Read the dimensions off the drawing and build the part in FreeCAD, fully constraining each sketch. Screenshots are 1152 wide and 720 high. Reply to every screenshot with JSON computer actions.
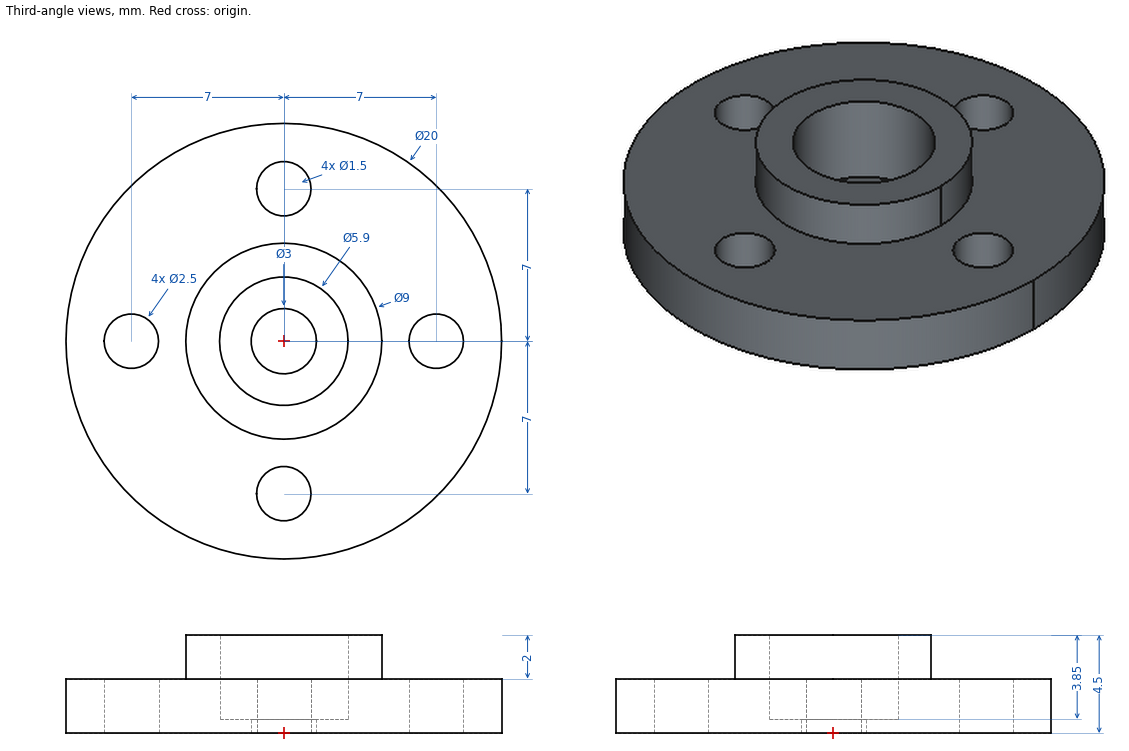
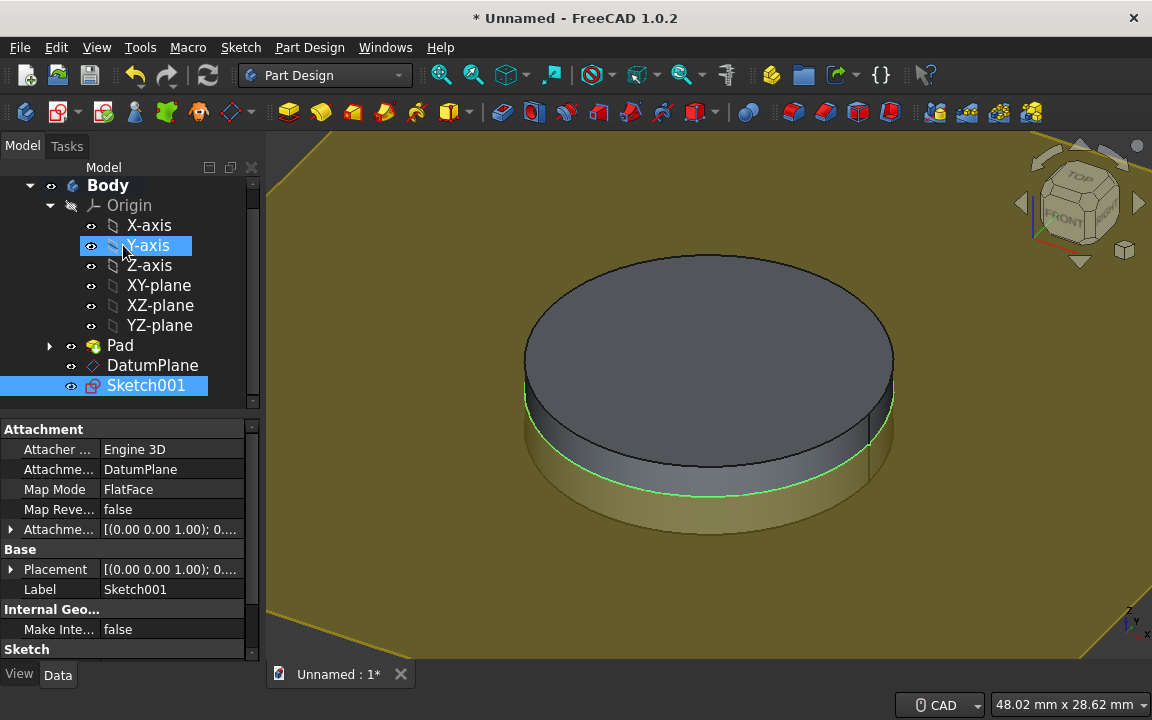
{"action": "left_click", "coordinate": [504, 112]}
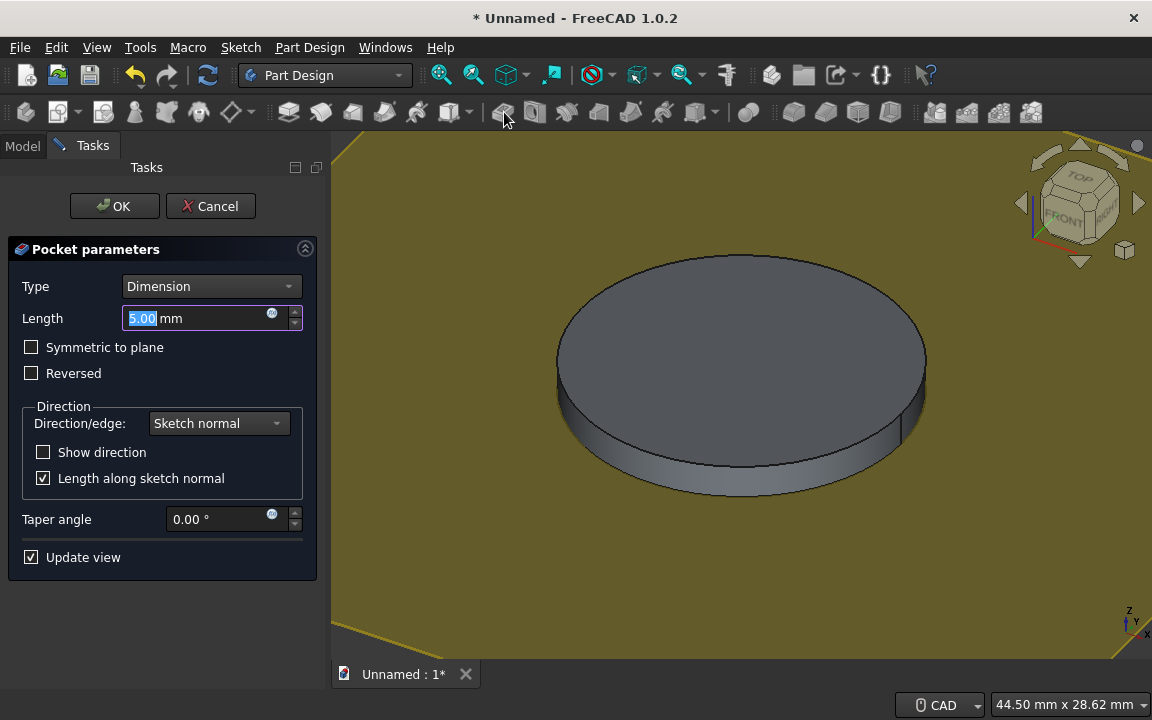
{"action": "type", "text": "2"}
{"action": "key", "text": "Tab"}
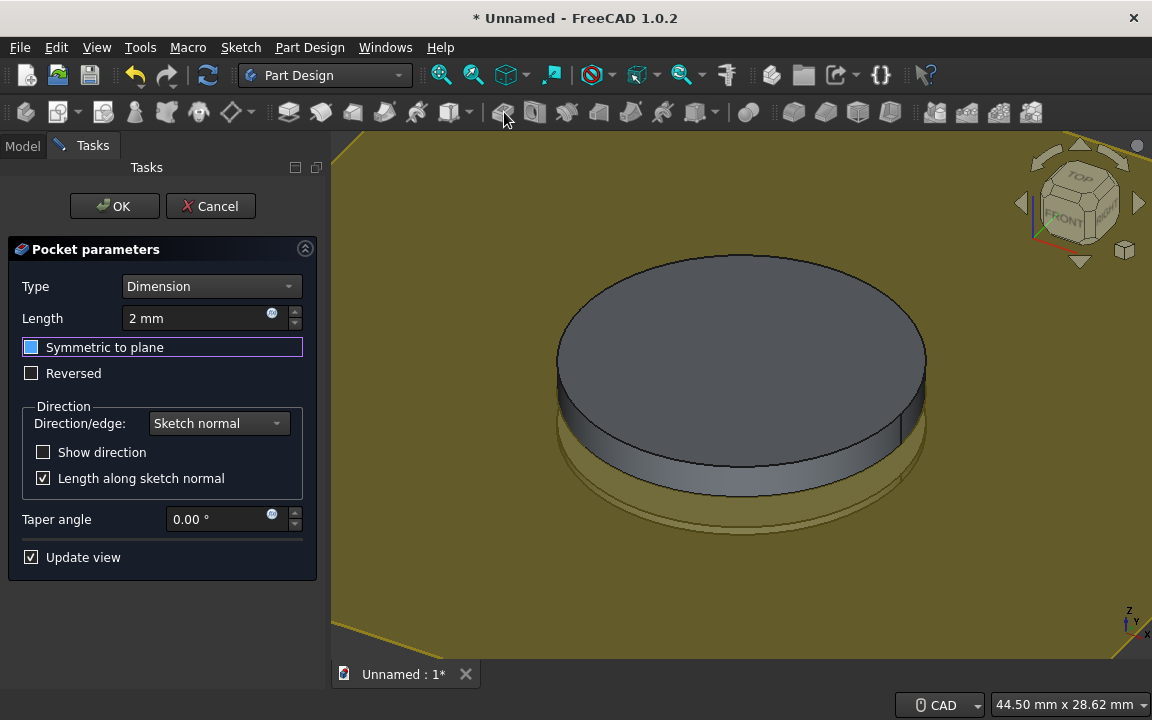
{"action": "left_click", "coordinate": [30, 373]}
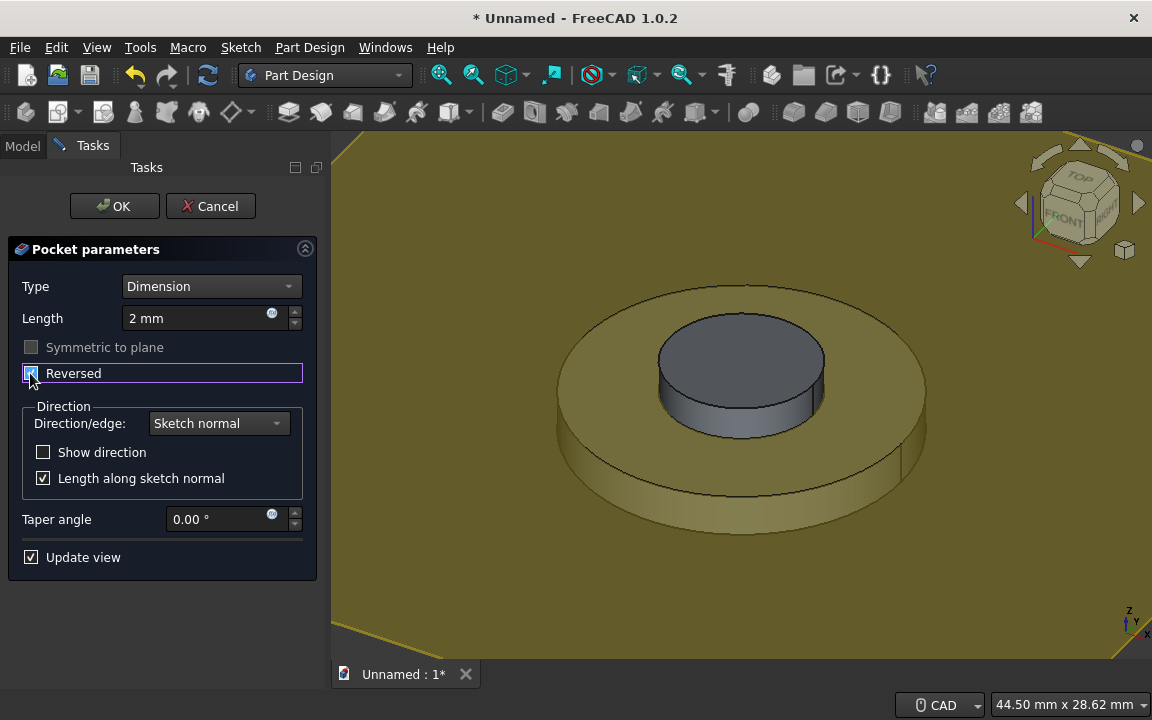
{"action": "left_click", "coordinate": [115, 206]}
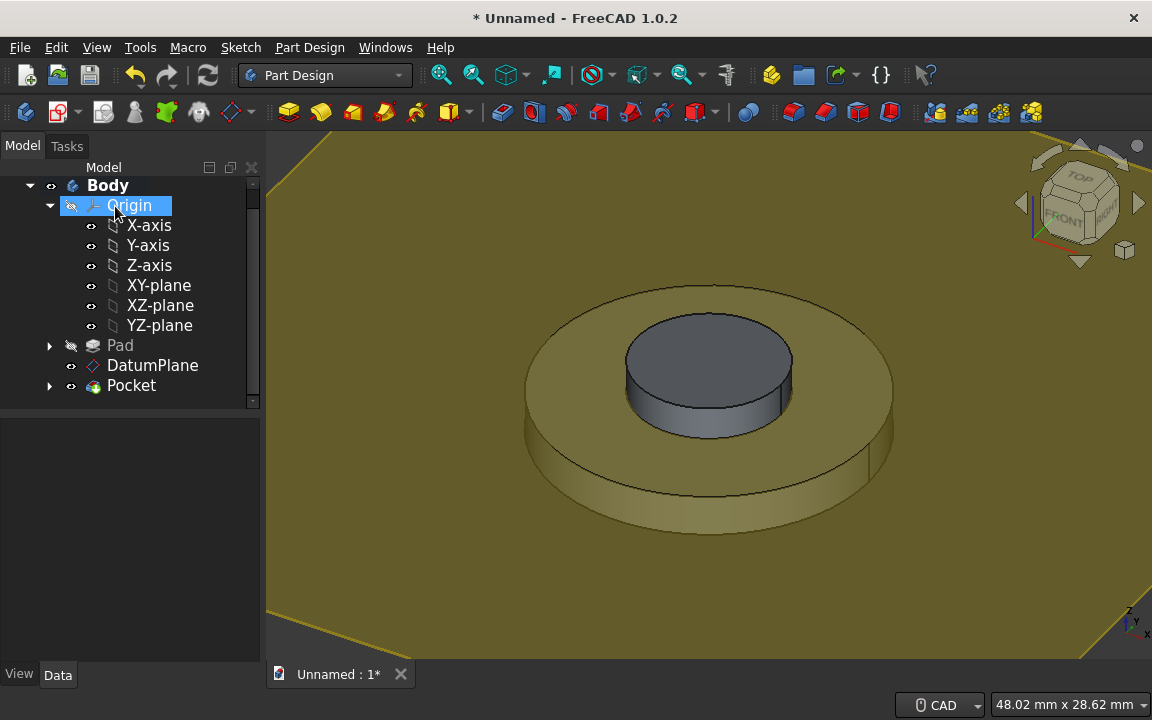
{"action": "left_click", "coordinate": [116, 366]}
{"action": "key", "text": "space"}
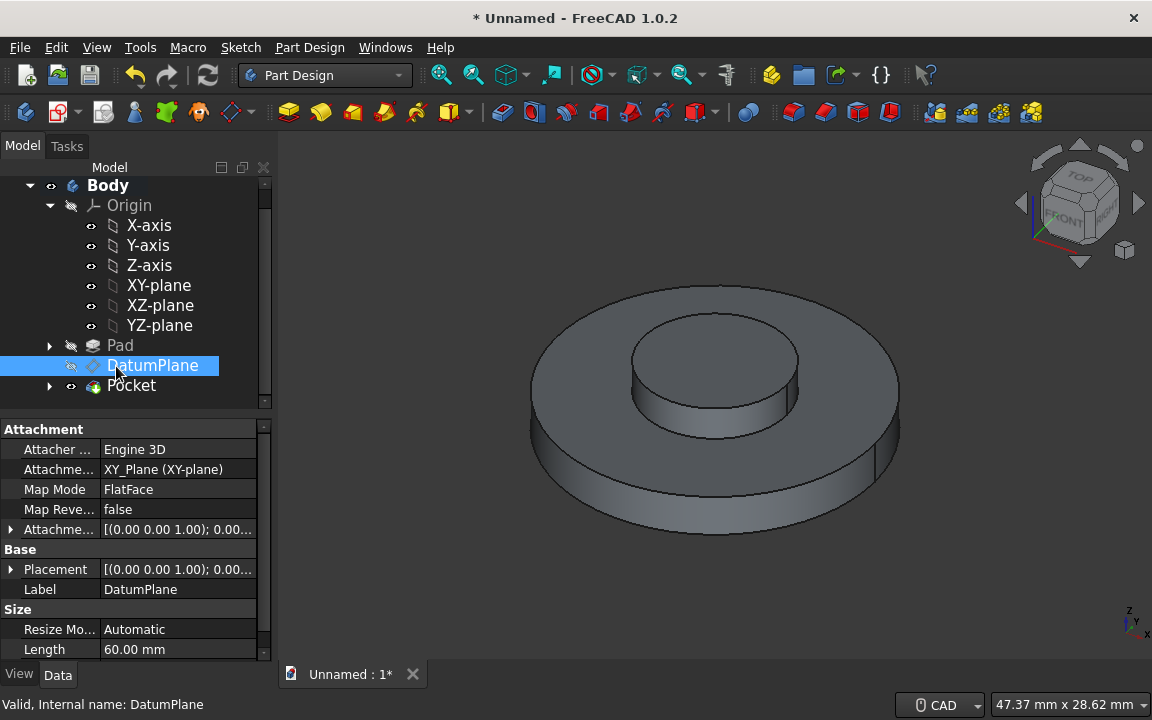
{"action": "left_click", "coordinate": [754, 473]}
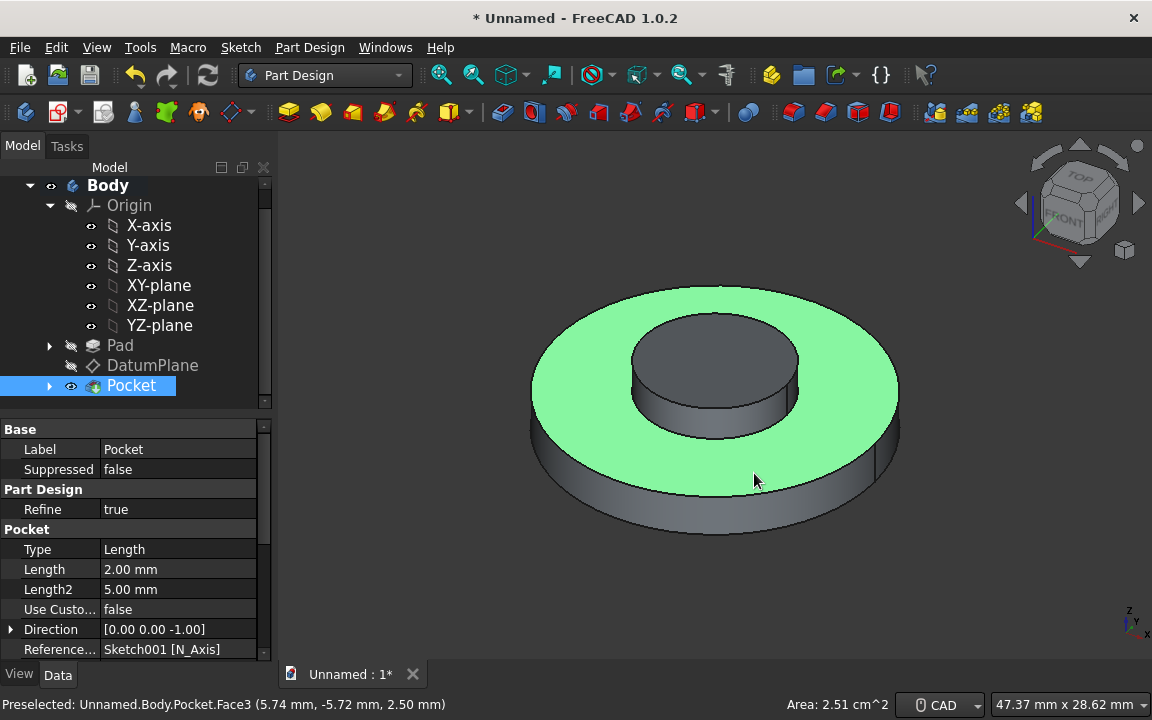
{"action": "left_click", "coordinate": [58, 112]}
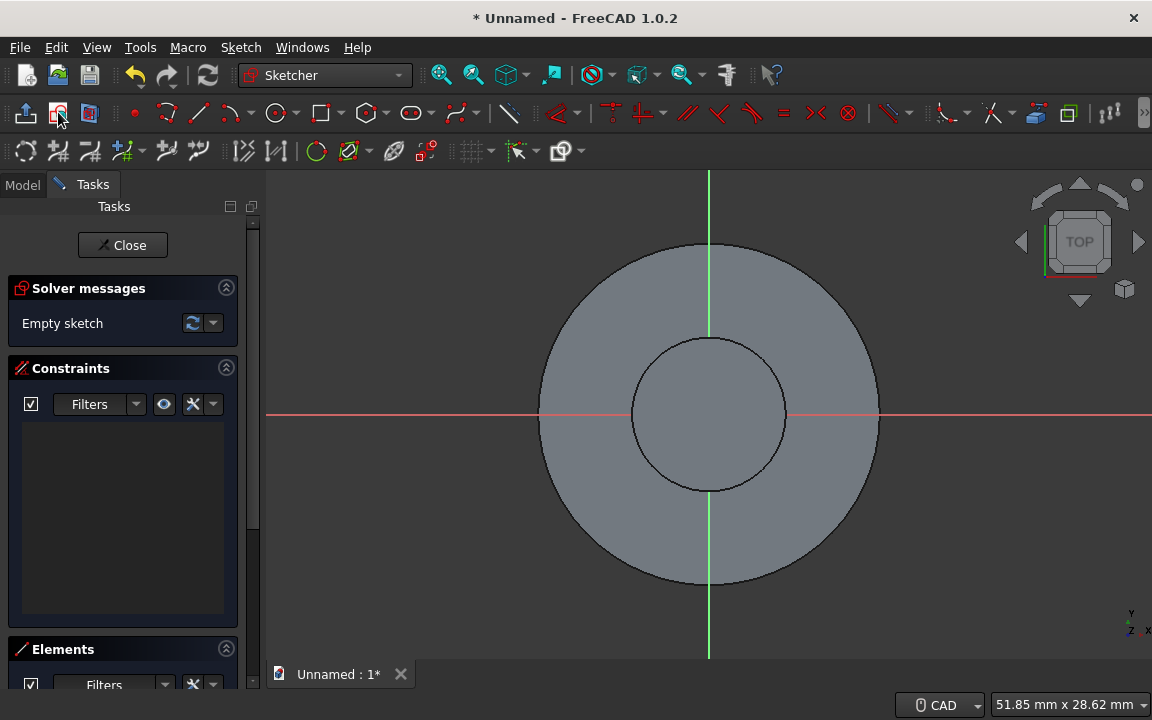
{"action": "key", "text": "g c"}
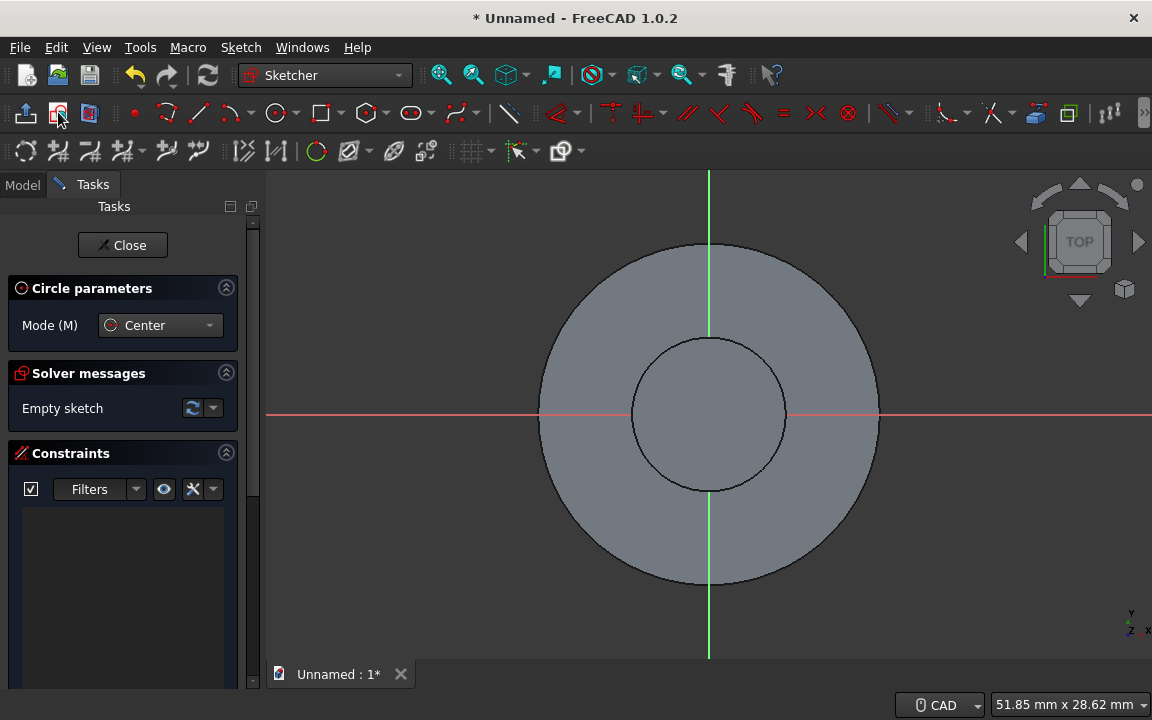
{"action": "scroll", "coordinate": [709, 295], "scroll_direction": "up", "scroll_amount": 3}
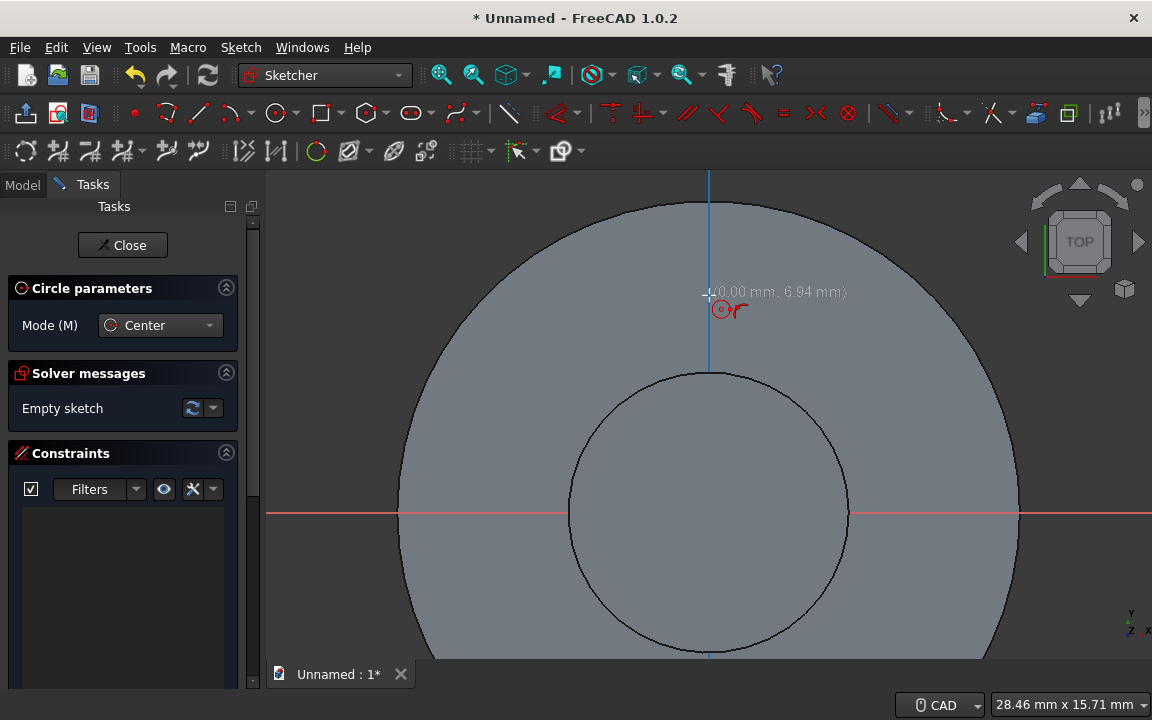
{"action": "left_click", "coordinate": [709, 295]}
{"action": "left_click", "coordinate": [725, 278]}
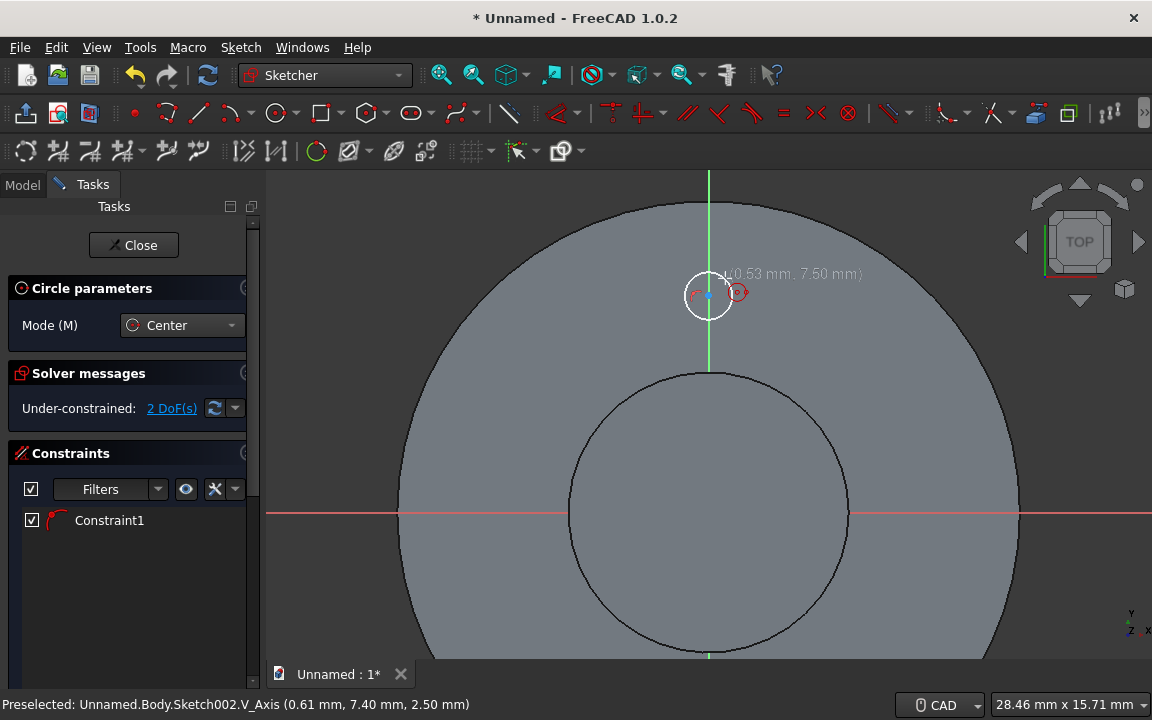
{"action": "left_click", "coordinate": [927, 513]}
{"action": "left_click", "coordinate": [943, 496]}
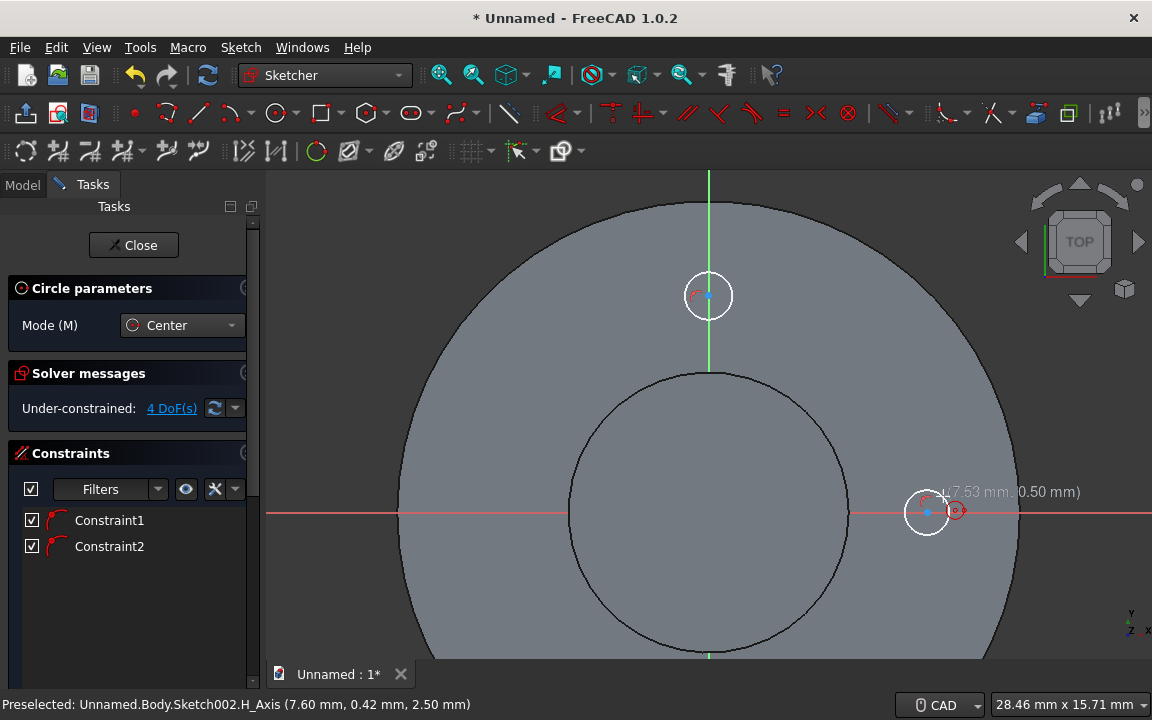
{"action": "scroll", "coordinate": [502, 215], "scroll_direction": "down", "scroll_amount": 2}